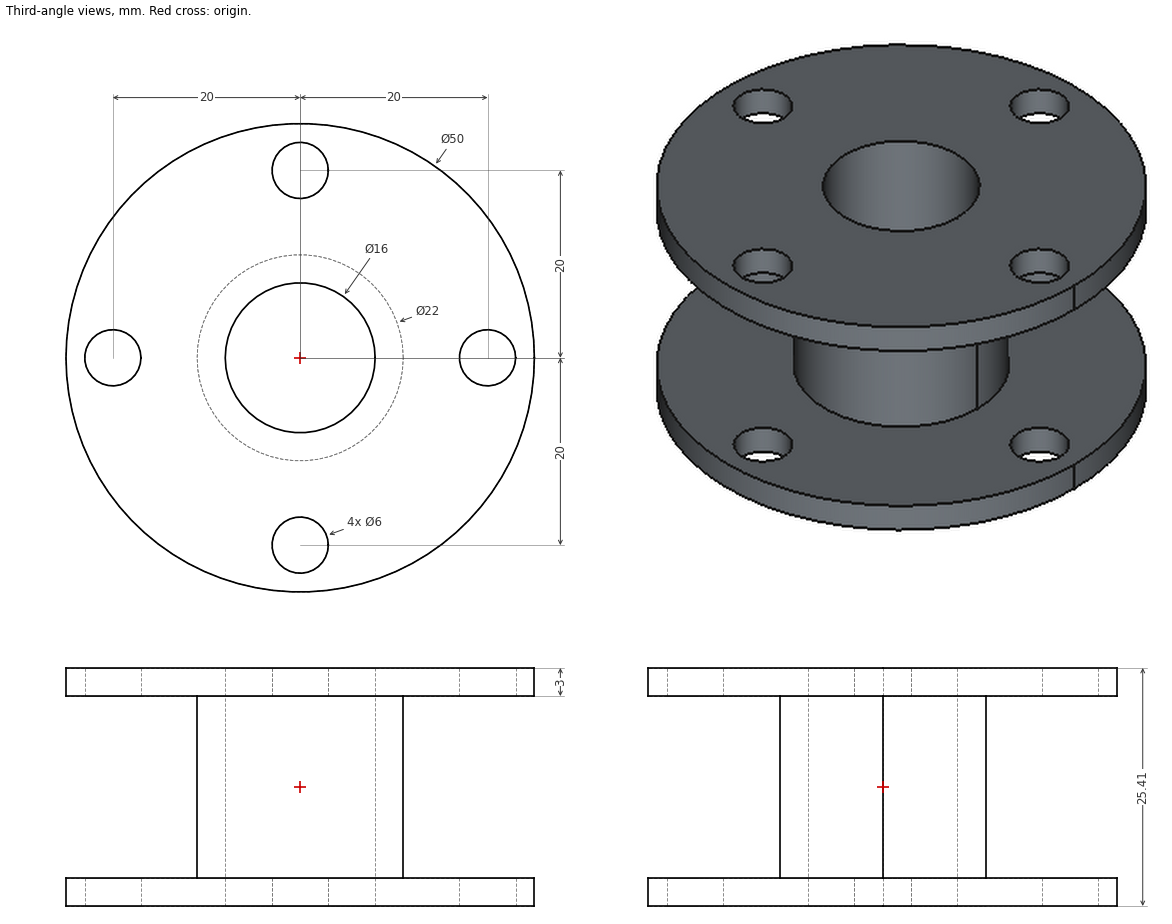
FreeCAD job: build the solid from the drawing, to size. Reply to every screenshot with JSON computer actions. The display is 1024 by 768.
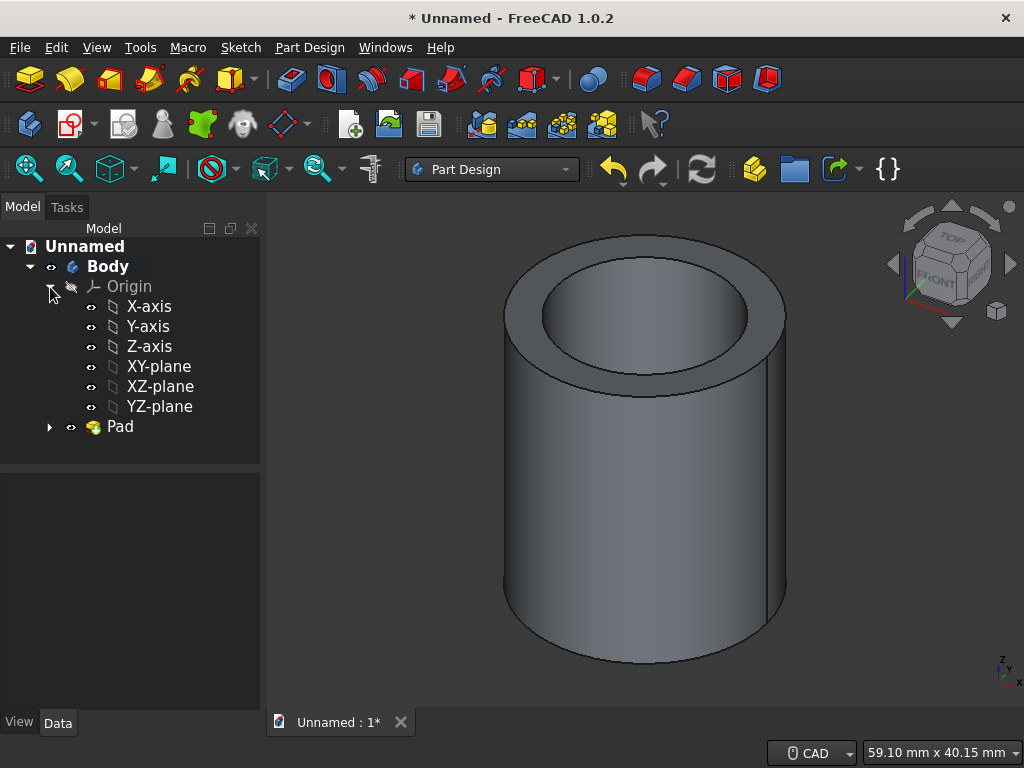
{"action": "left_click", "coordinate": [136, 367]}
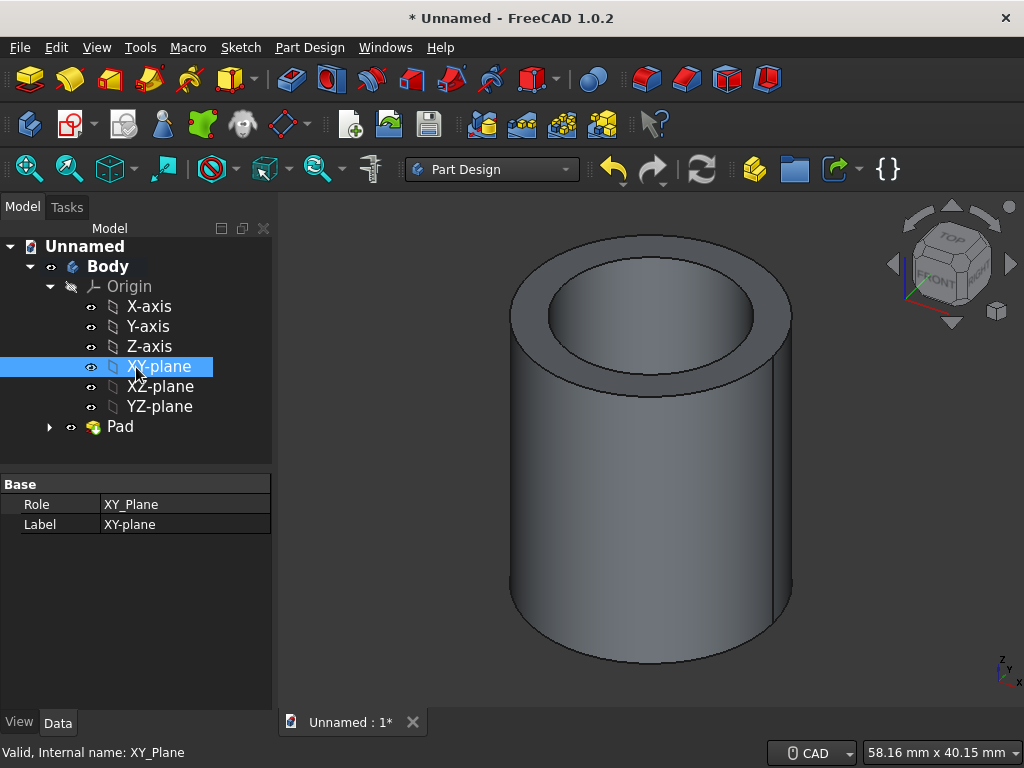
{"action": "left_click", "coordinate": [284, 124]}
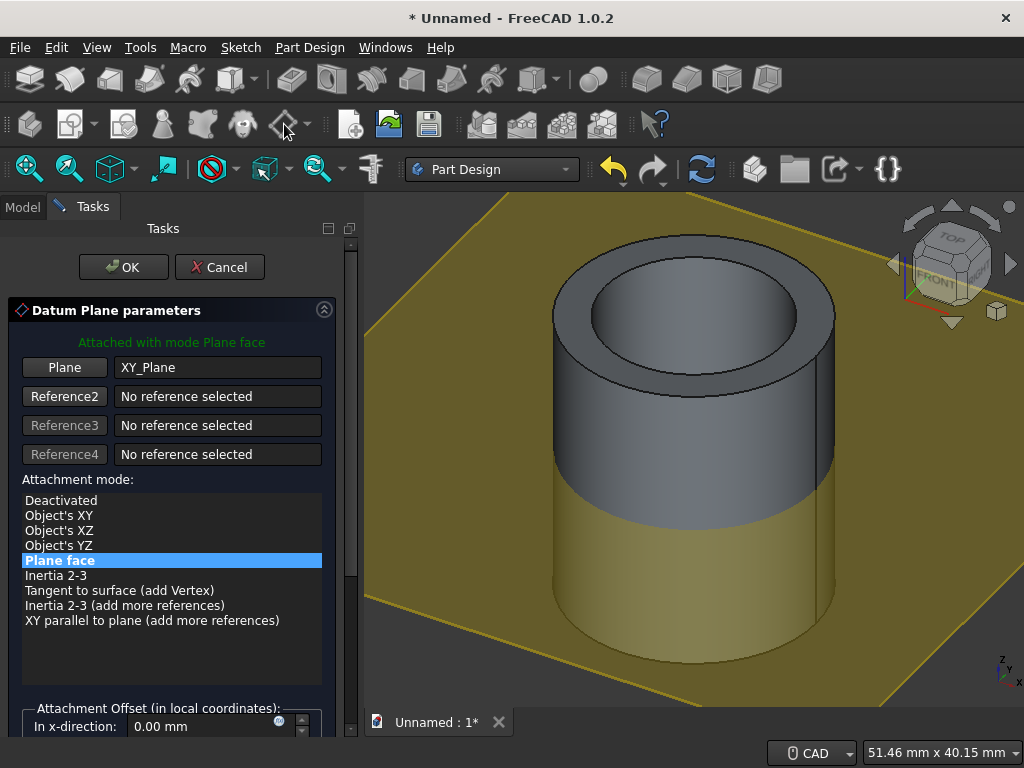
{"action": "scroll", "coordinate": [351, 487], "scroll_direction": "down", "scroll_amount": 3}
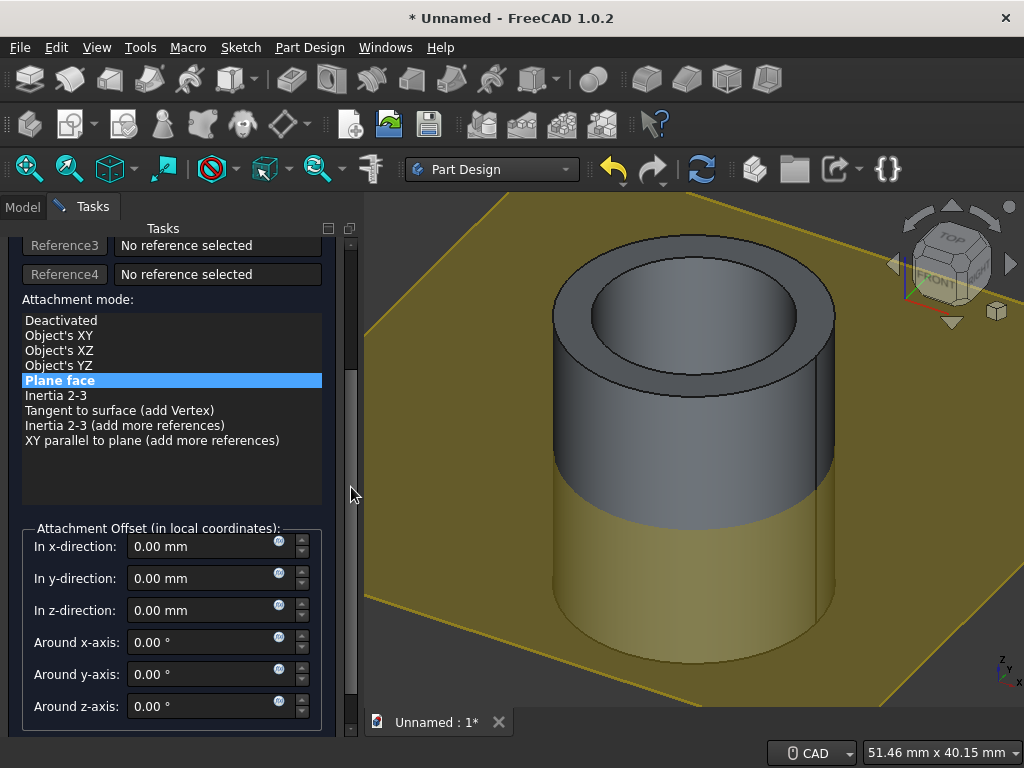
{"action": "triple_click", "coordinate": [210, 610]}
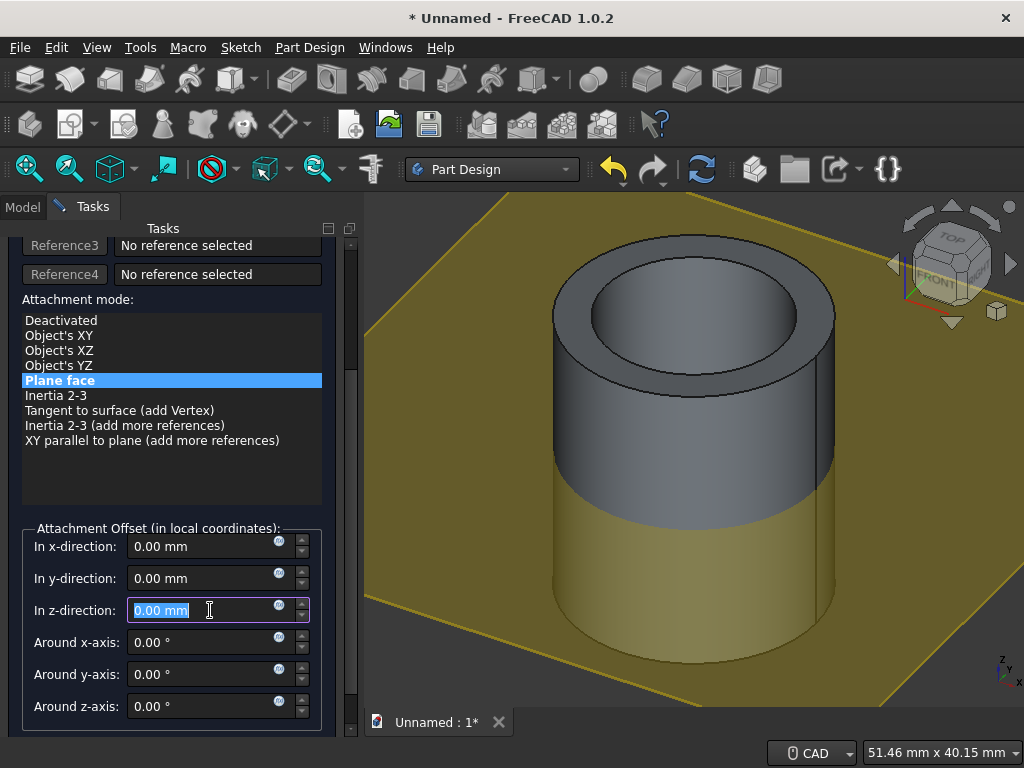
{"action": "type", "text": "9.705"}
{"action": "key", "text": "Tab"}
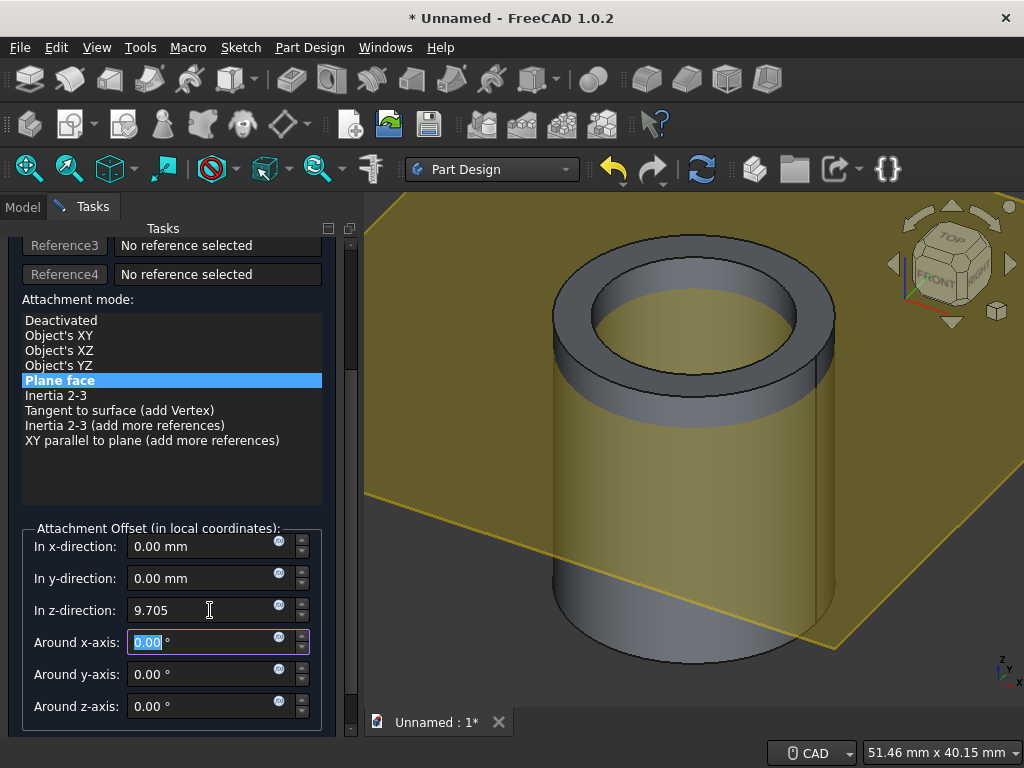
{"action": "scroll", "coordinate": [351, 487], "scroll_direction": "up", "scroll_amount": 4}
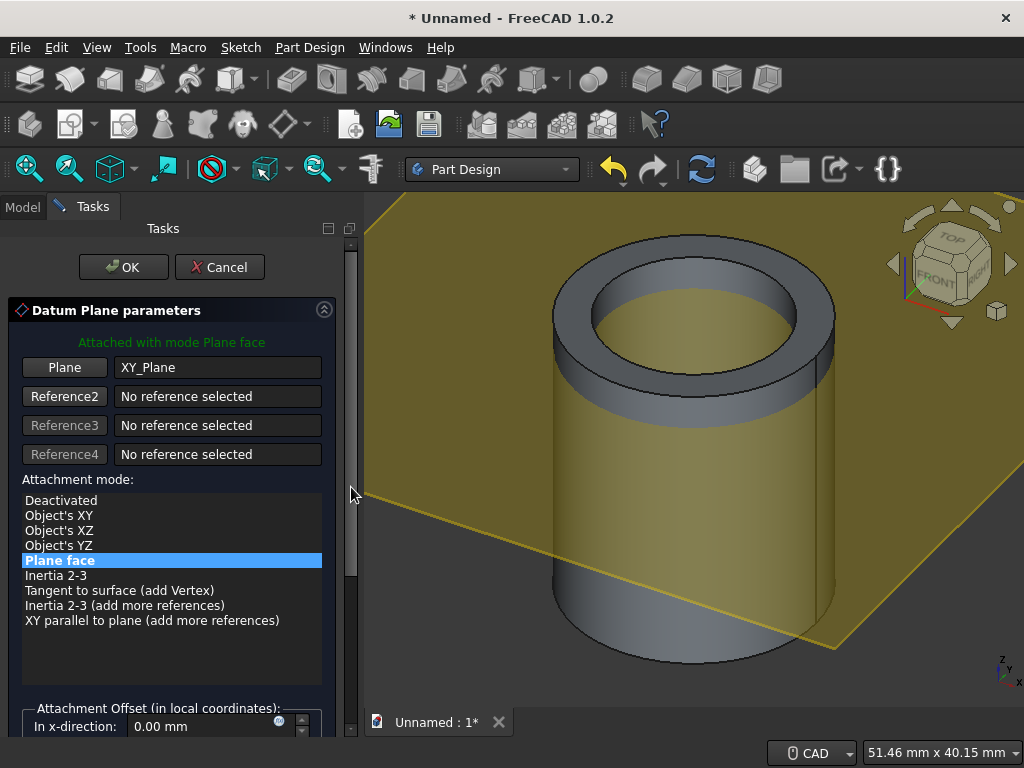
{"action": "left_click", "coordinate": [124, 267]}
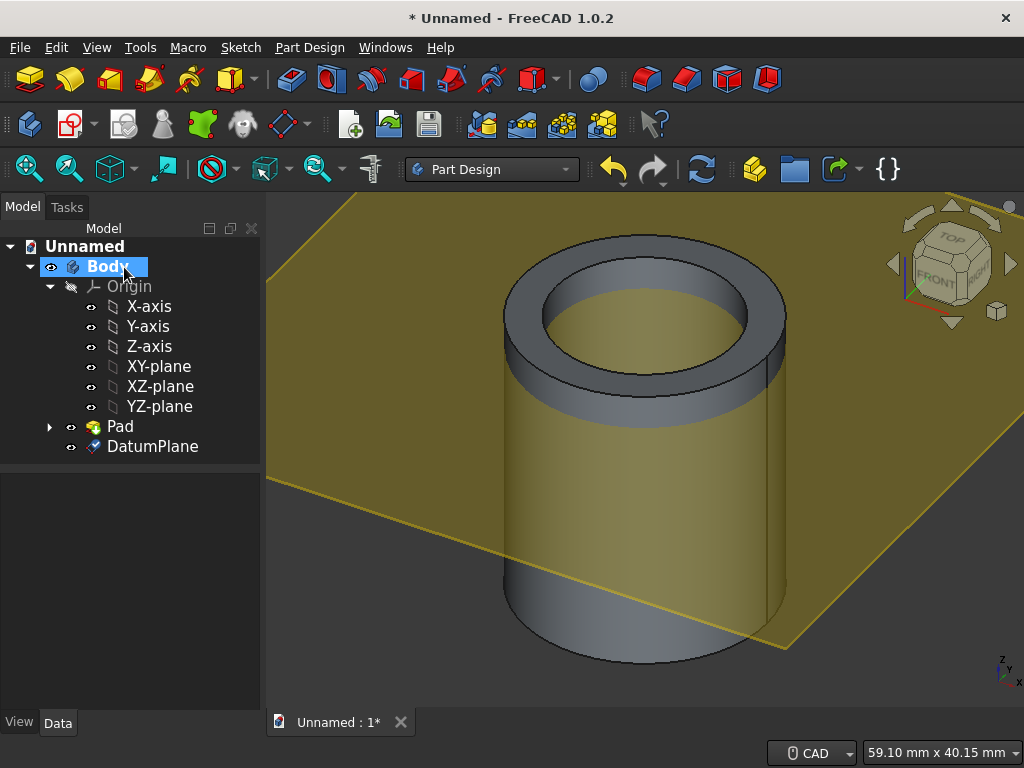
{"action": "left_click", "coordinate": [116, 447]}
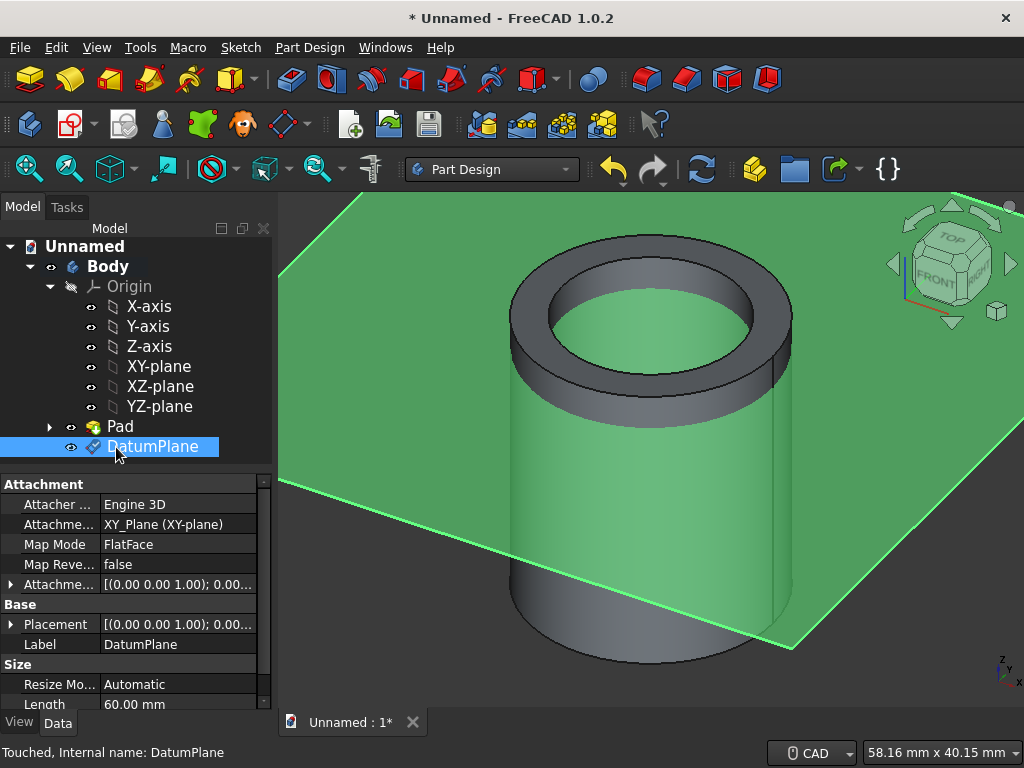
{"action": "left_click", "coordinate": [70, 124]}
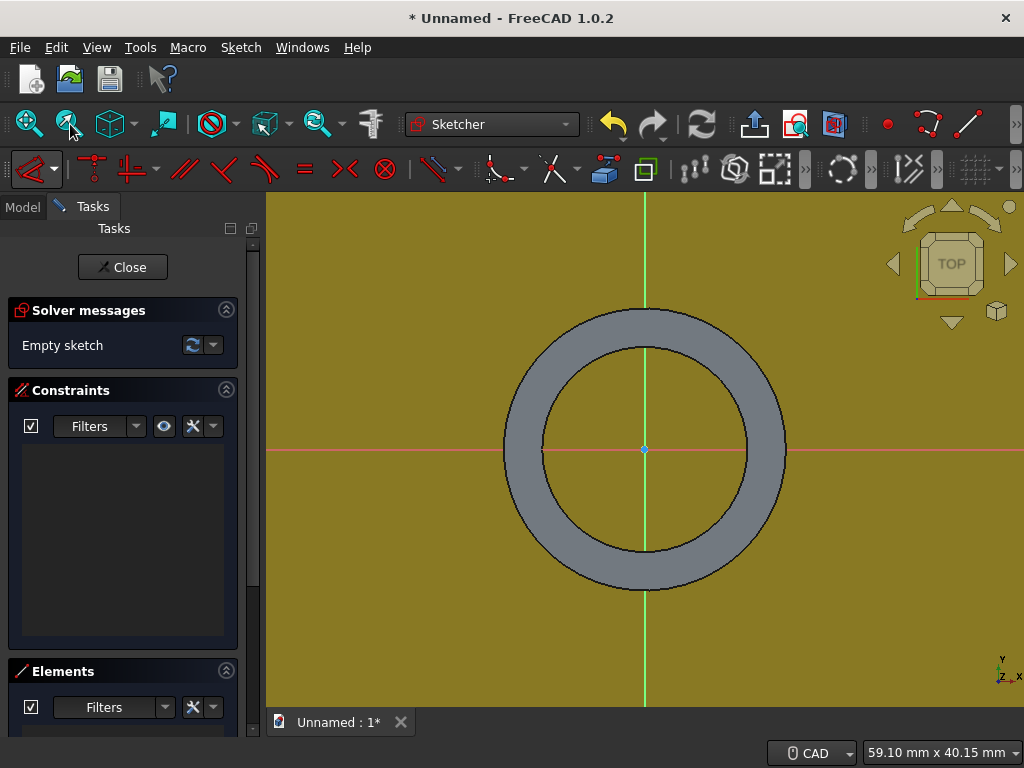
{"action": "left_click", "coordinate": [836, 124]}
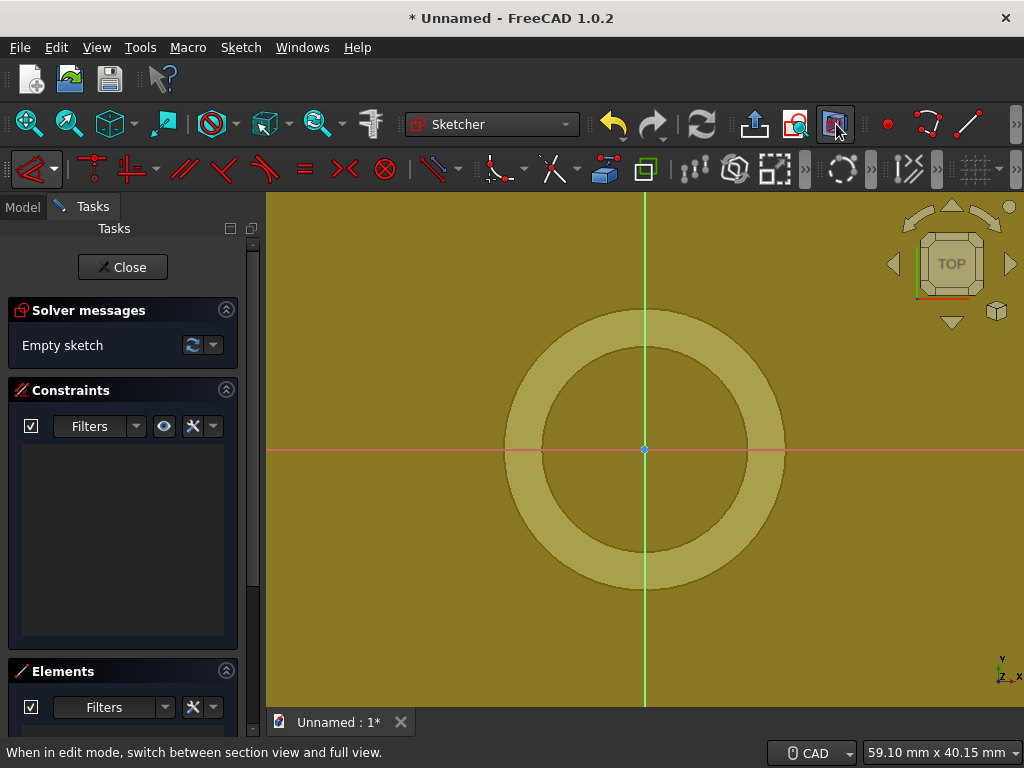
{"action": "scroll", "coordinate": [493, 450], "scroll_direction": "down", "scroll_amount": 3}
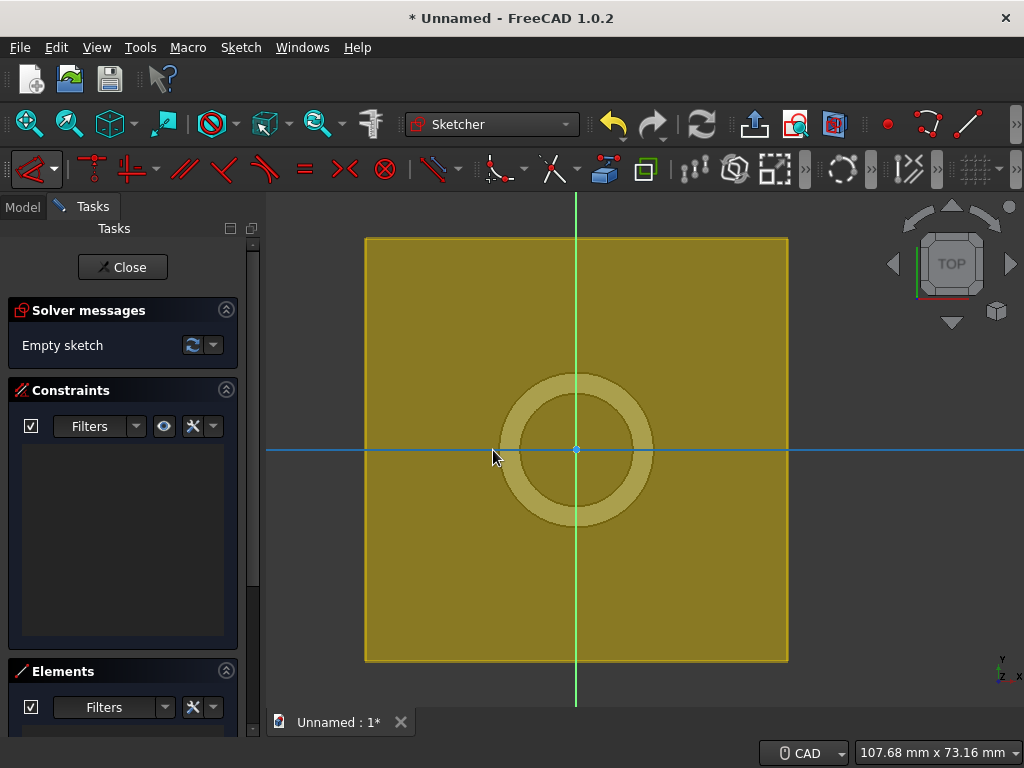
{"action": "key", "text": "g c"}